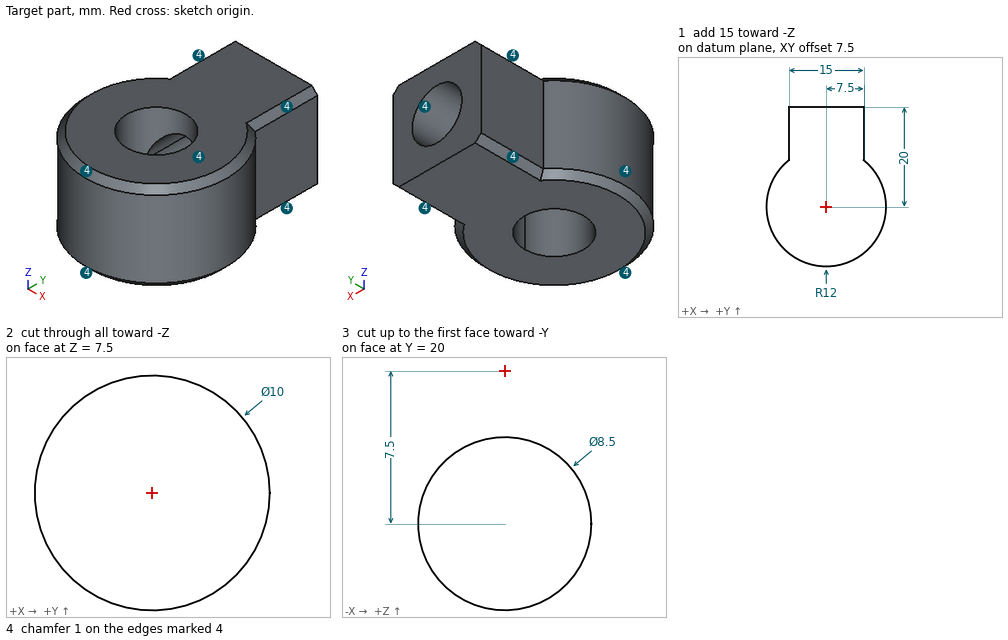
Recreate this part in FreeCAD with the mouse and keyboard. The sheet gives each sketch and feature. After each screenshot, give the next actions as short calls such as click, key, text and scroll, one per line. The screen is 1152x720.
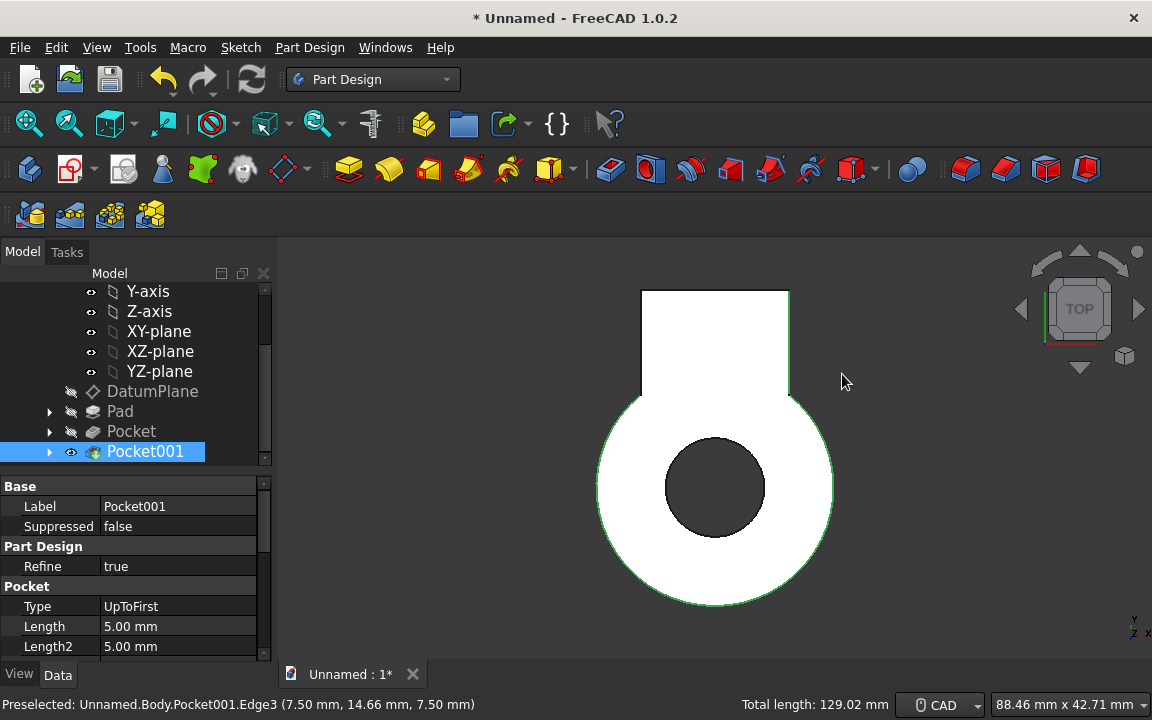
click(641, 341, ctrl)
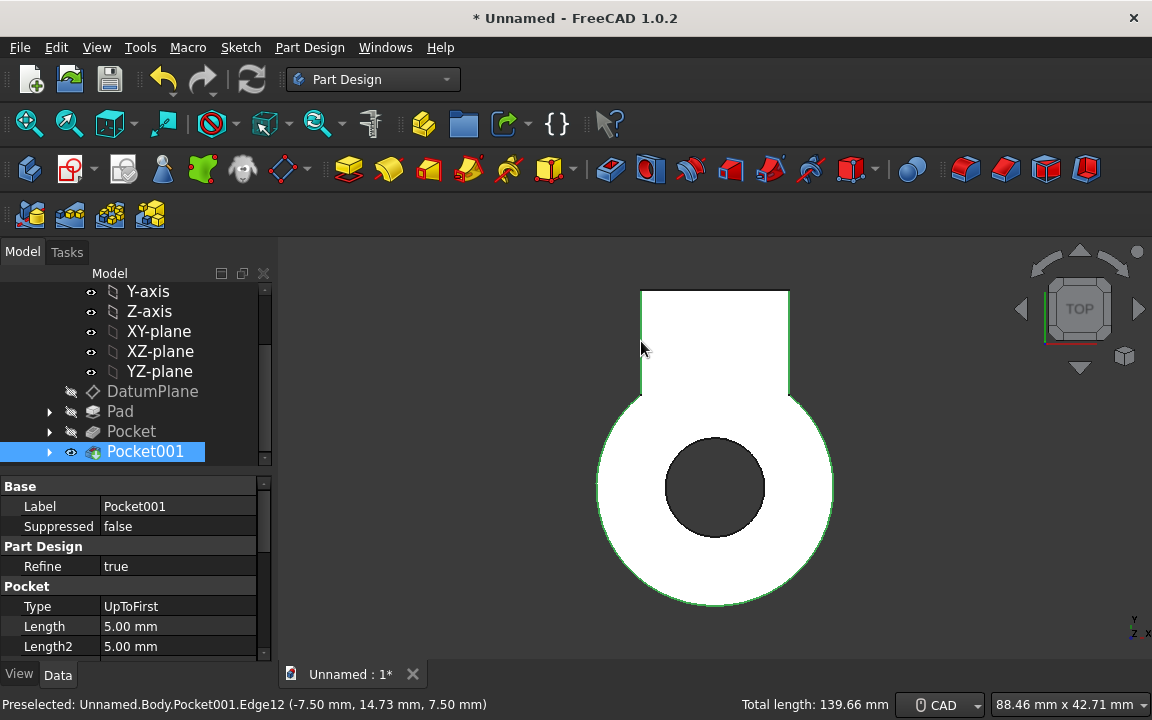
key(1)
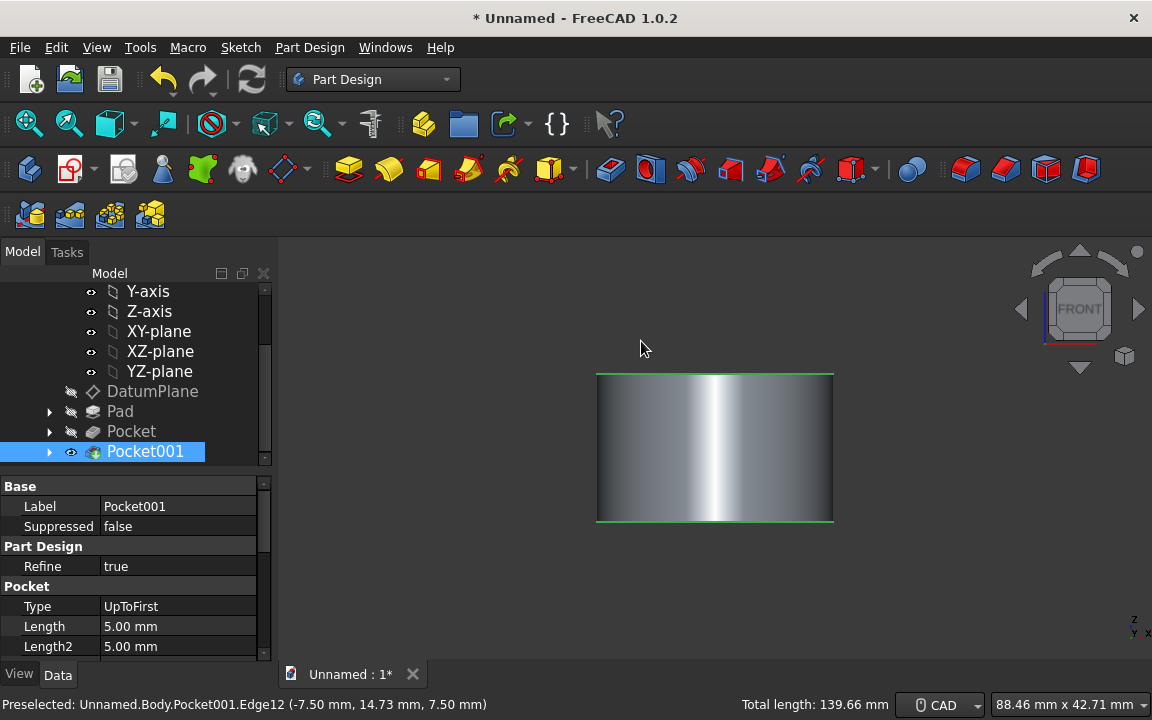
click(30, 124)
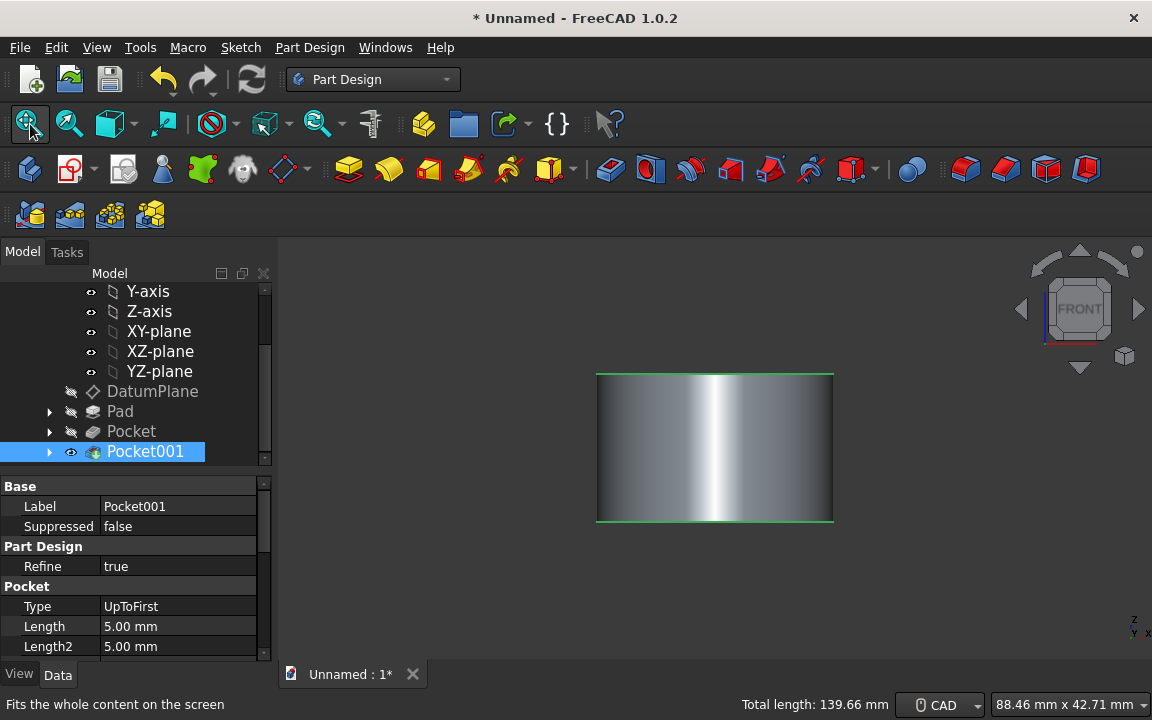
key(3)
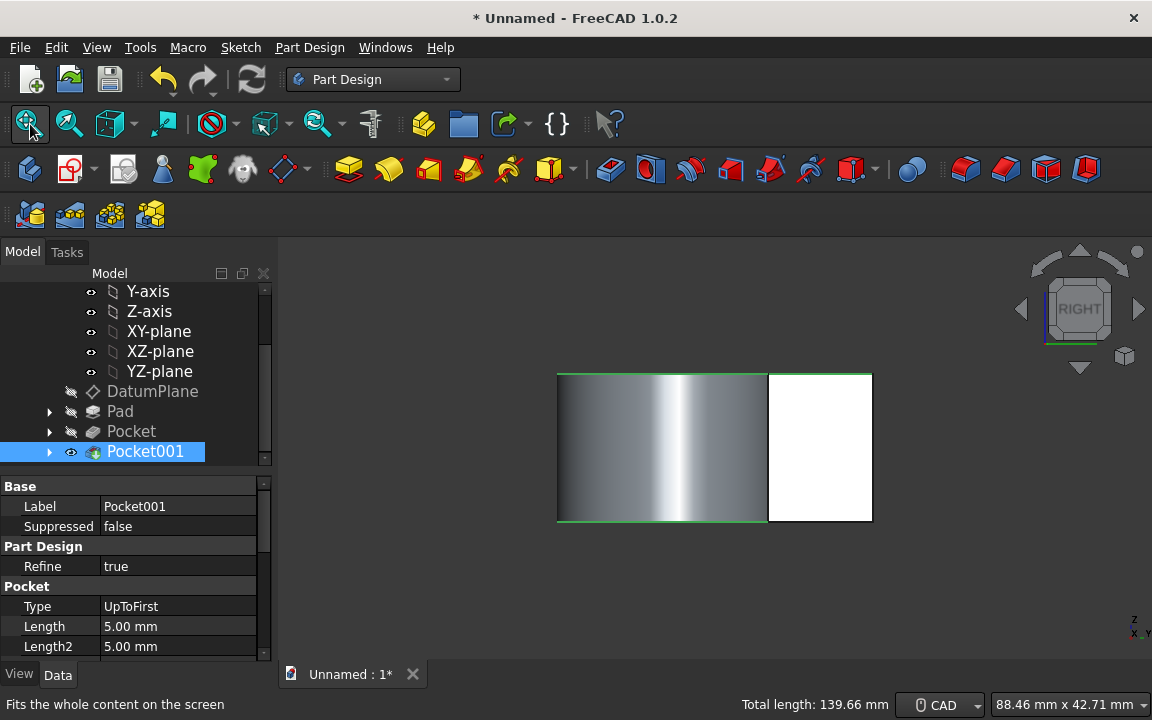
click(30, 124)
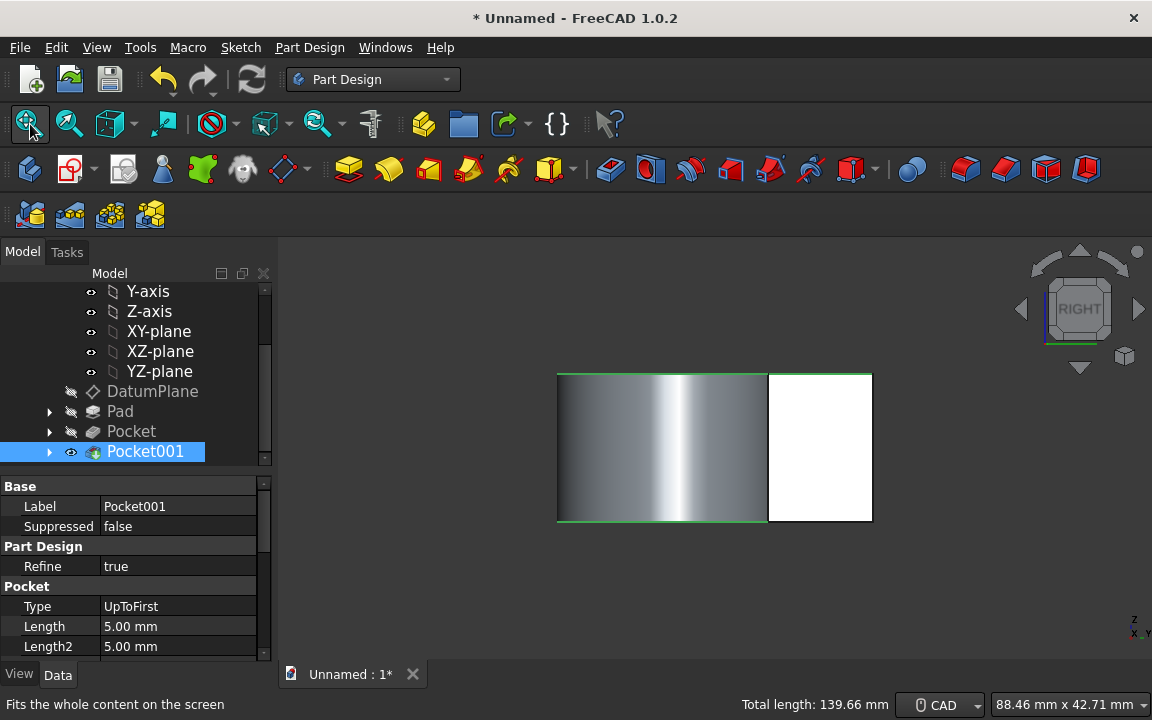
click(821, 521, ctrl)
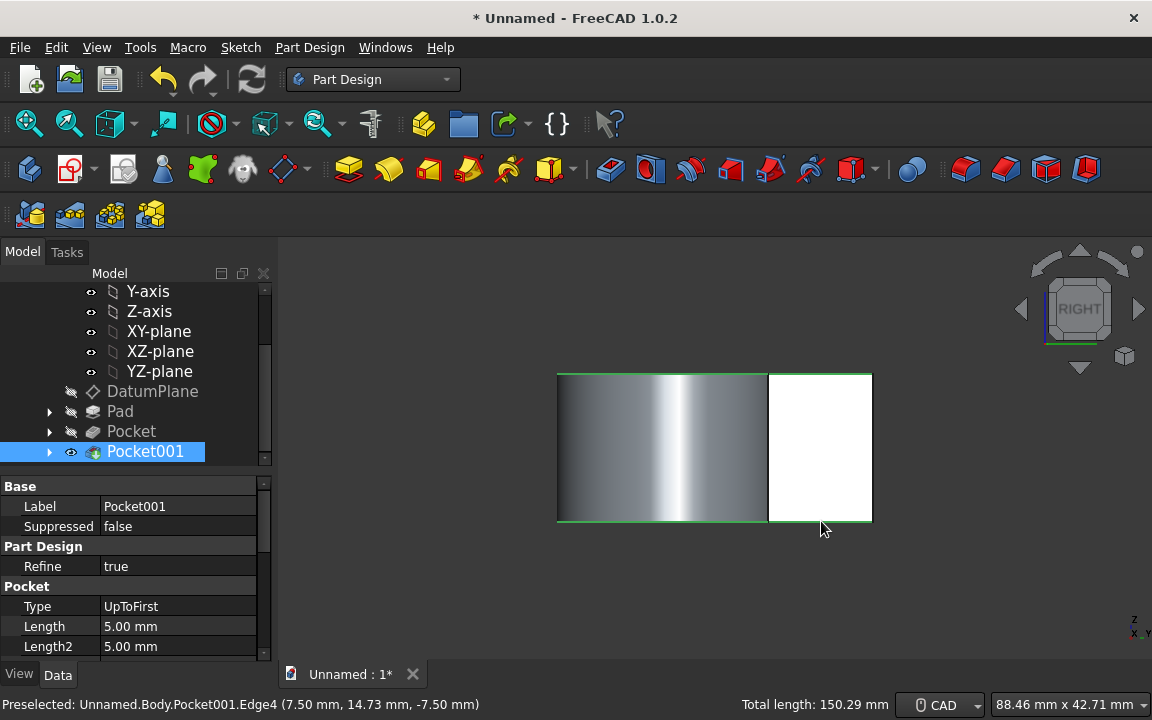
key(5)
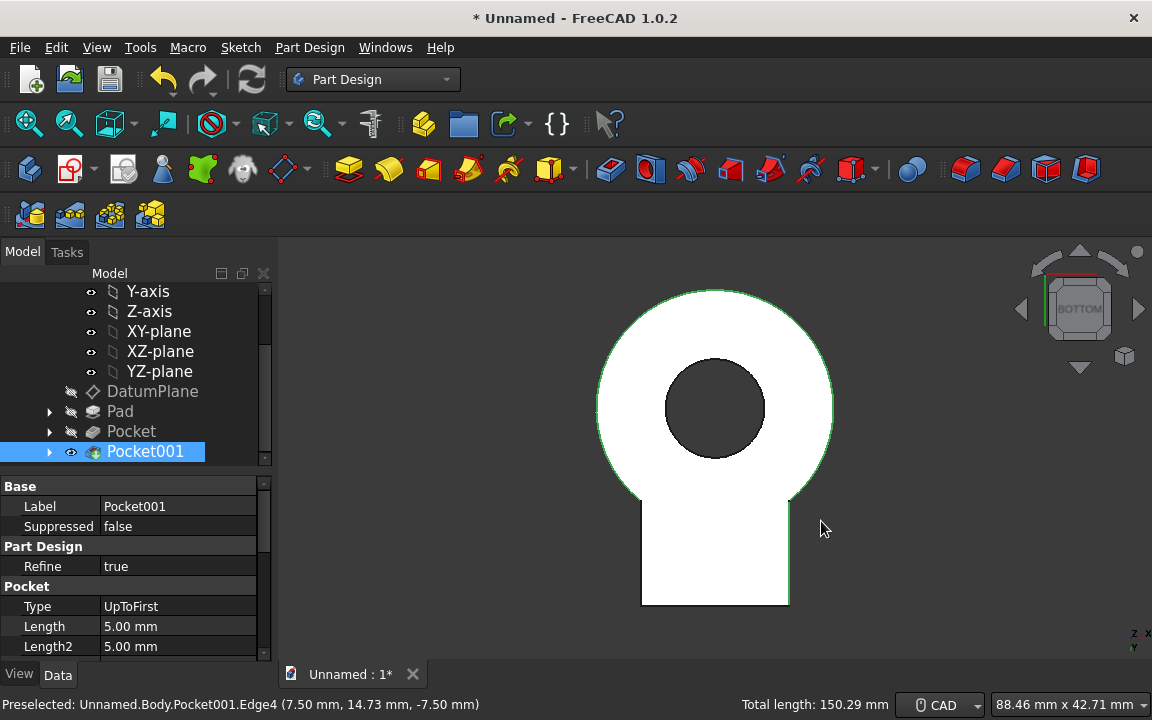
click(641, 553, ctrl)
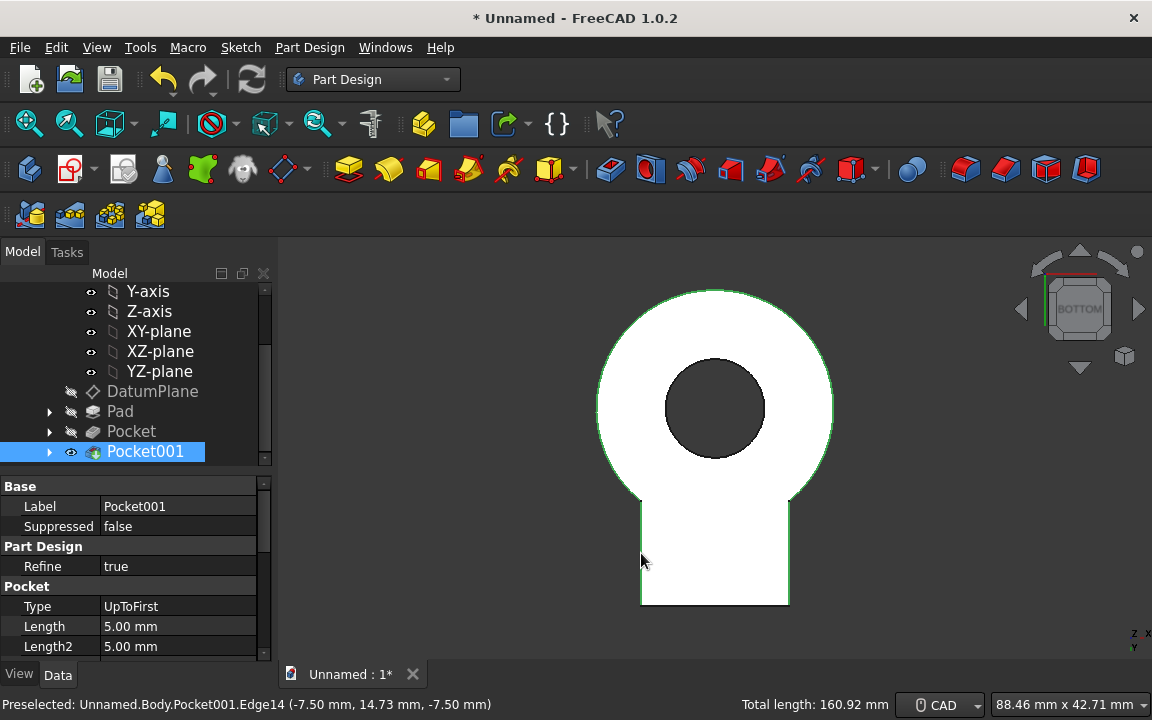
click(1006, 170)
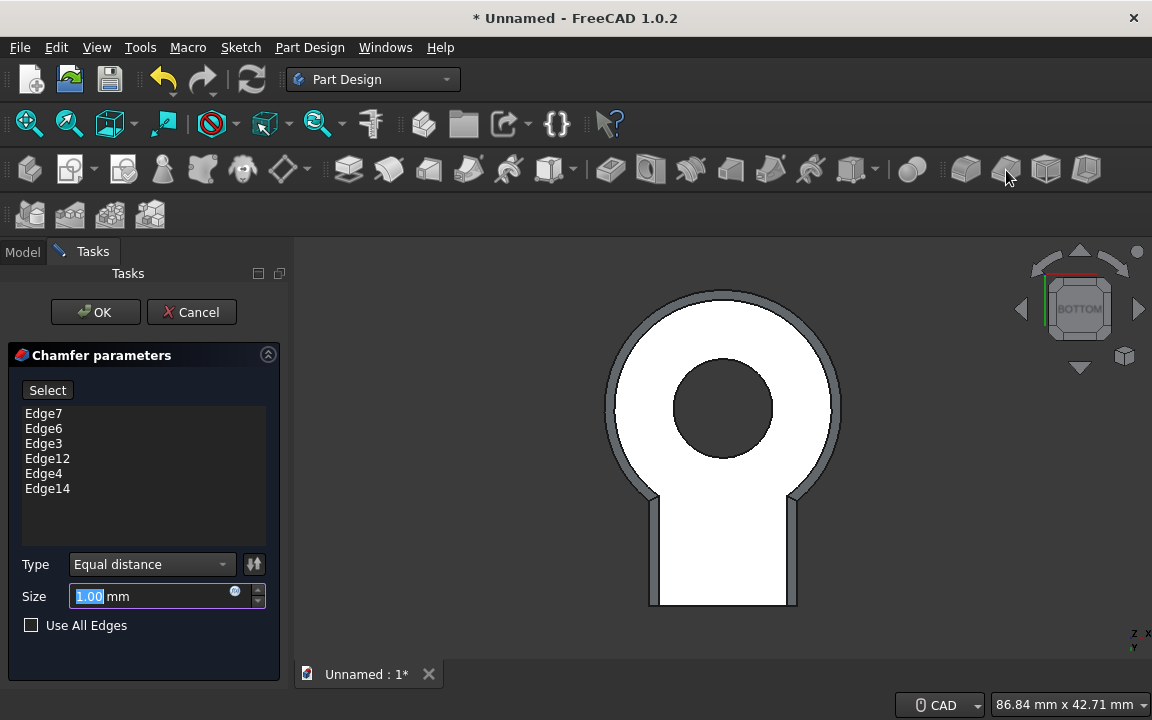
text(1)
key(Tab)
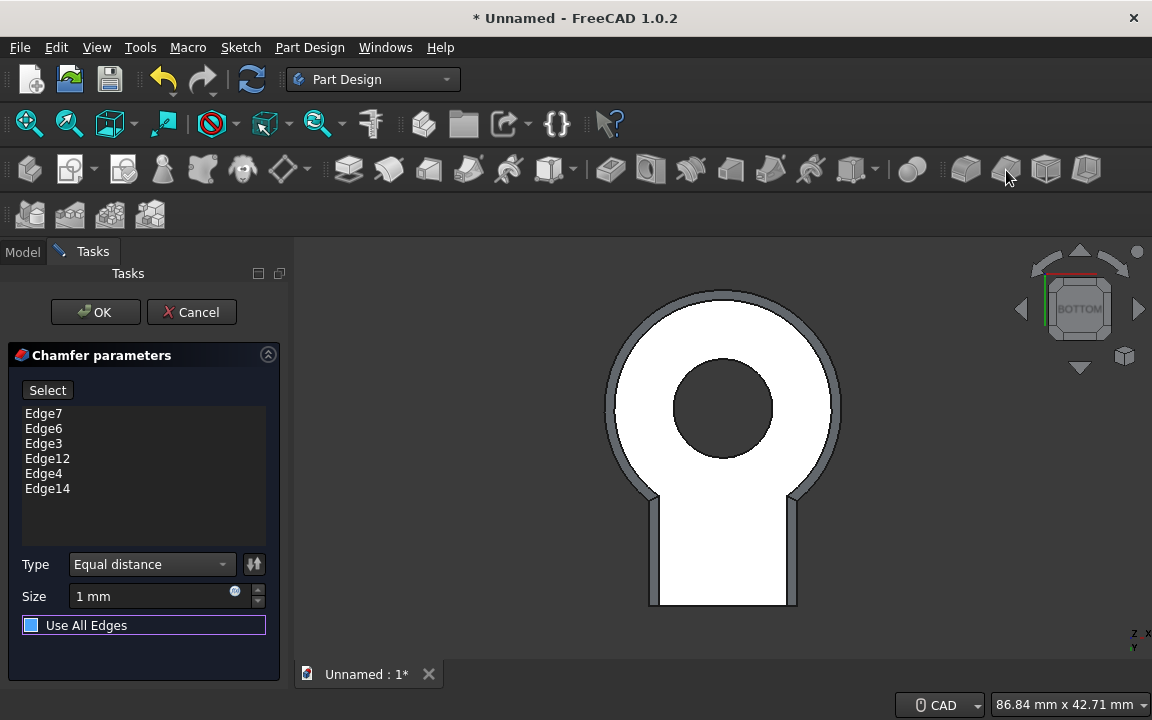
click(96, 312)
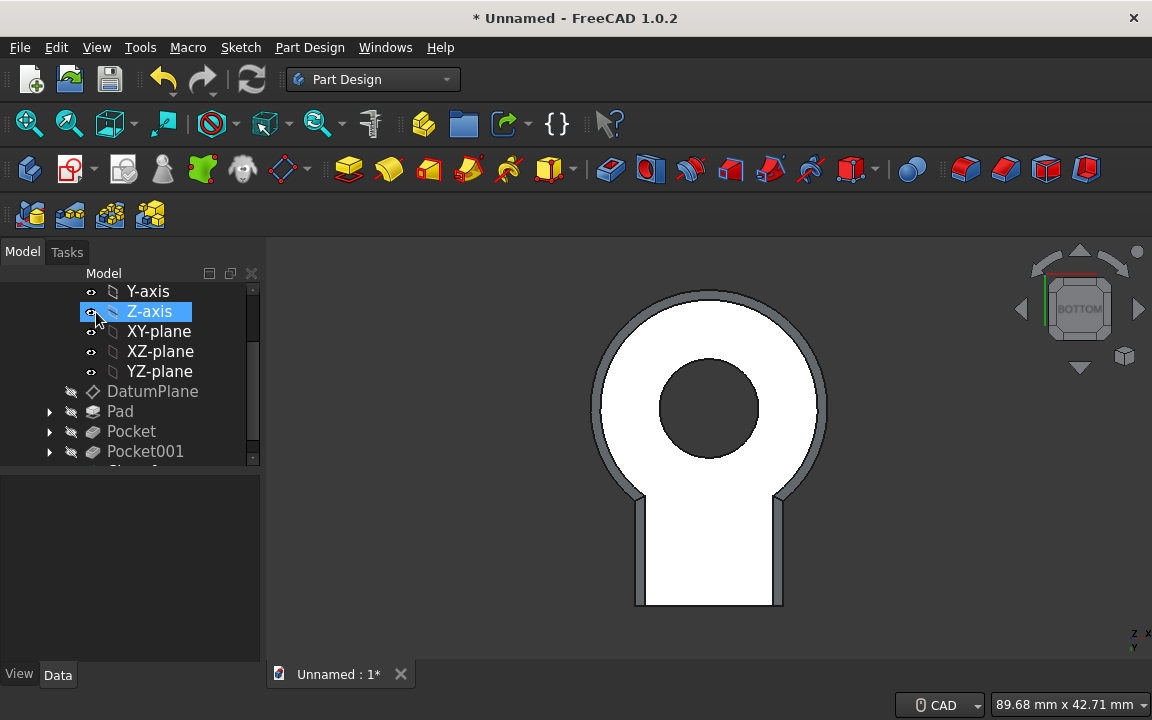
key(0)